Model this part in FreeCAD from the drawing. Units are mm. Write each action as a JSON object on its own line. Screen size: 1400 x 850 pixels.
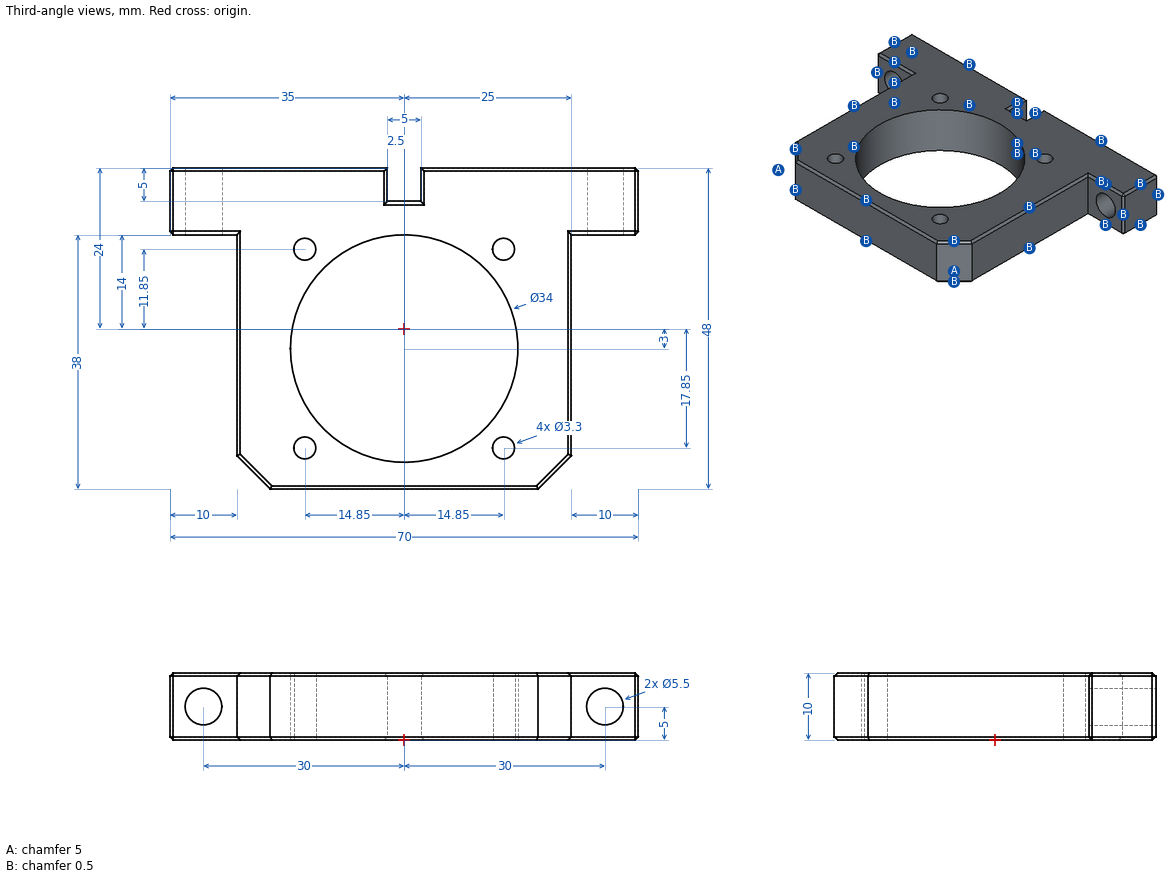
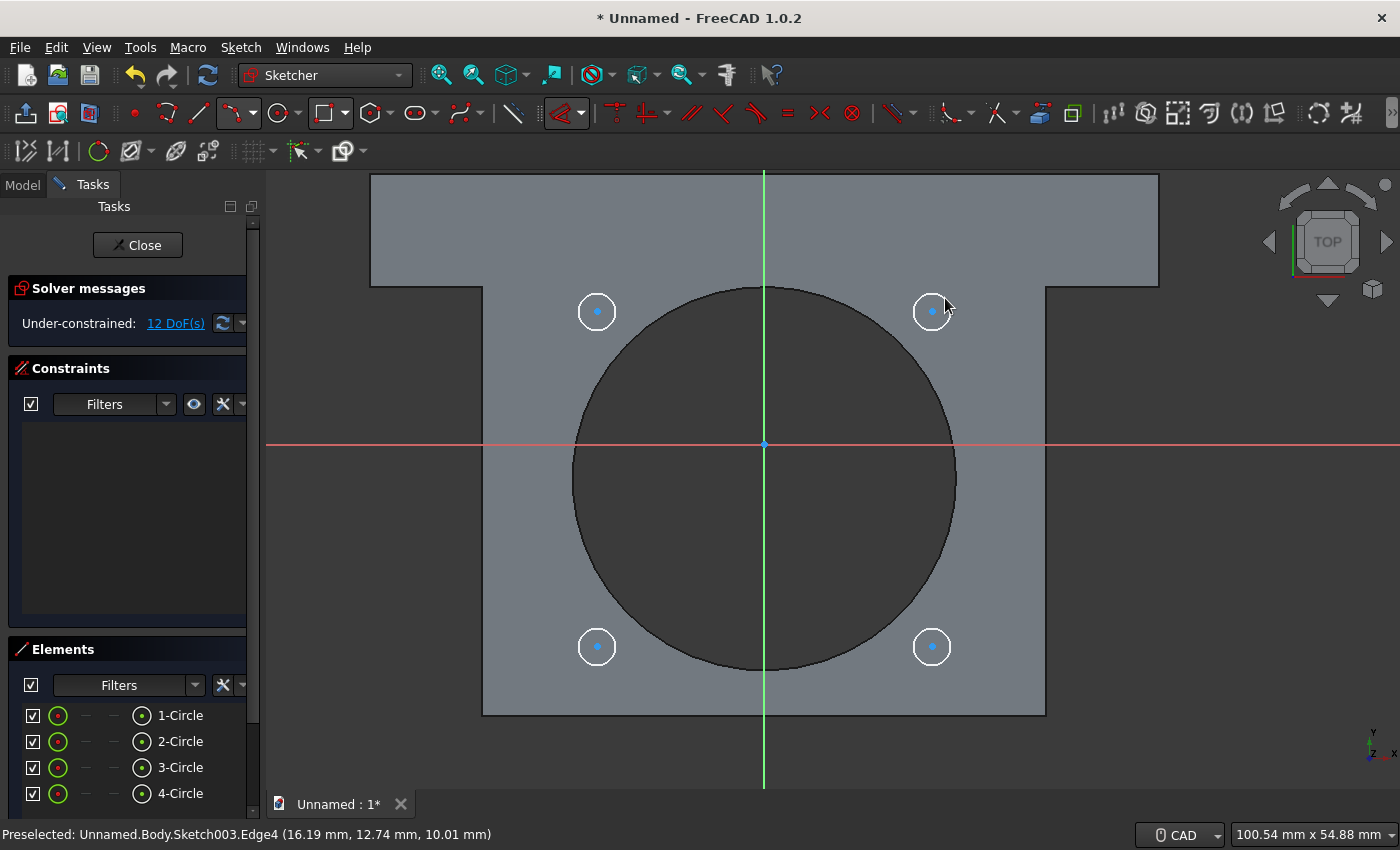
{"action": "left_click", "coordinate": [945, 634]}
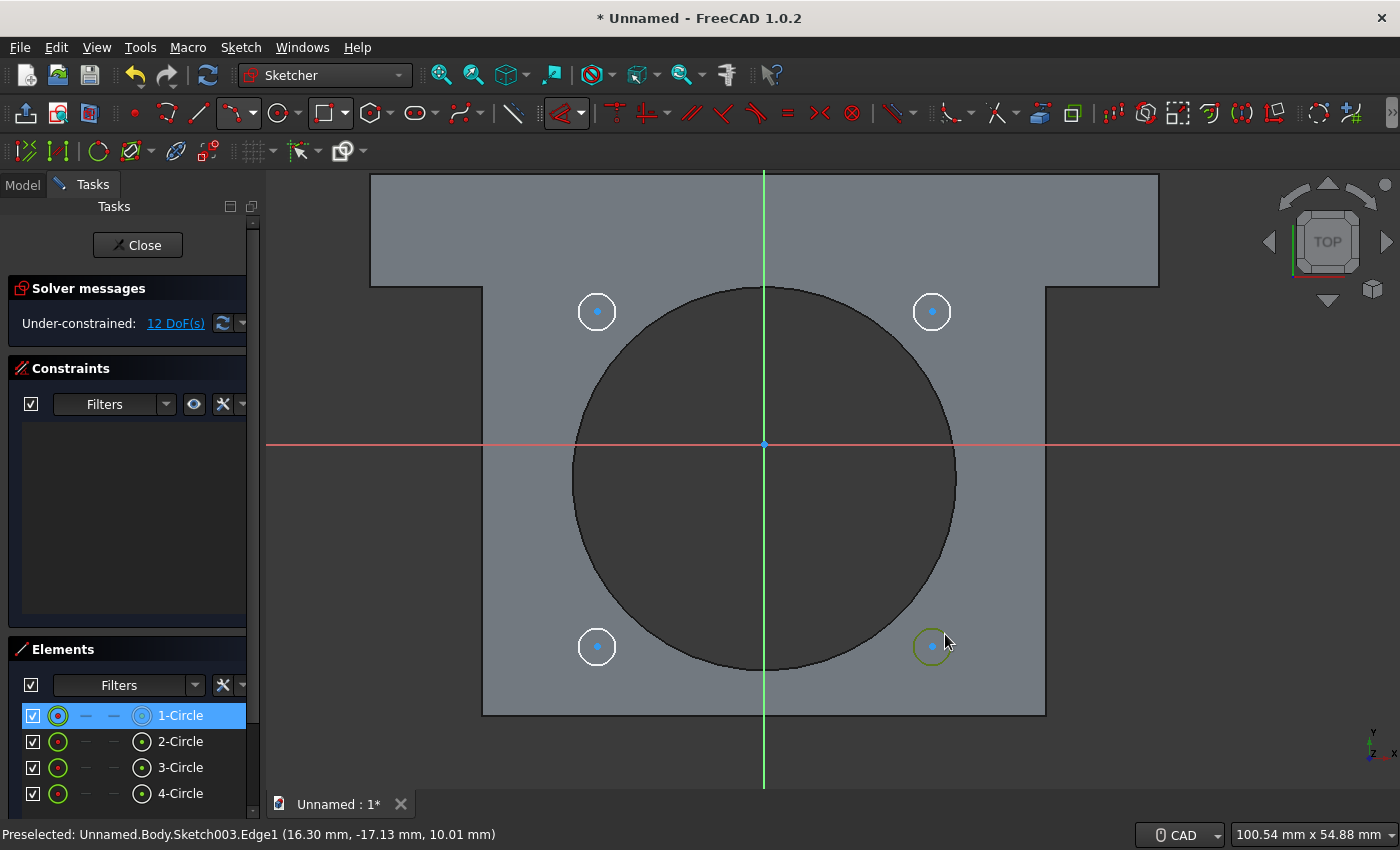
{"action": "left_click", "coordinate": [610, 634]}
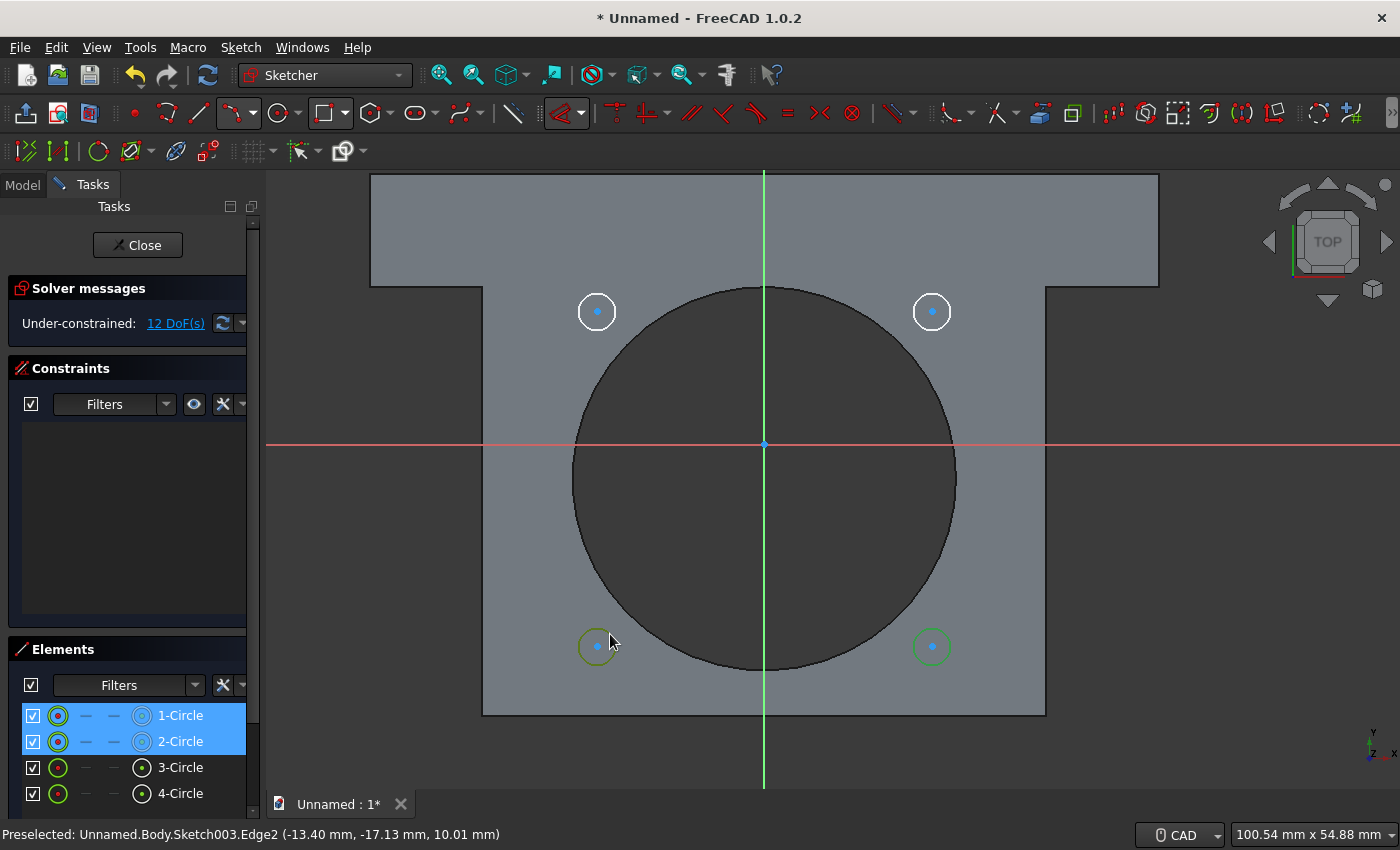
{"action": "left_click", "coordinate": [610, 299]}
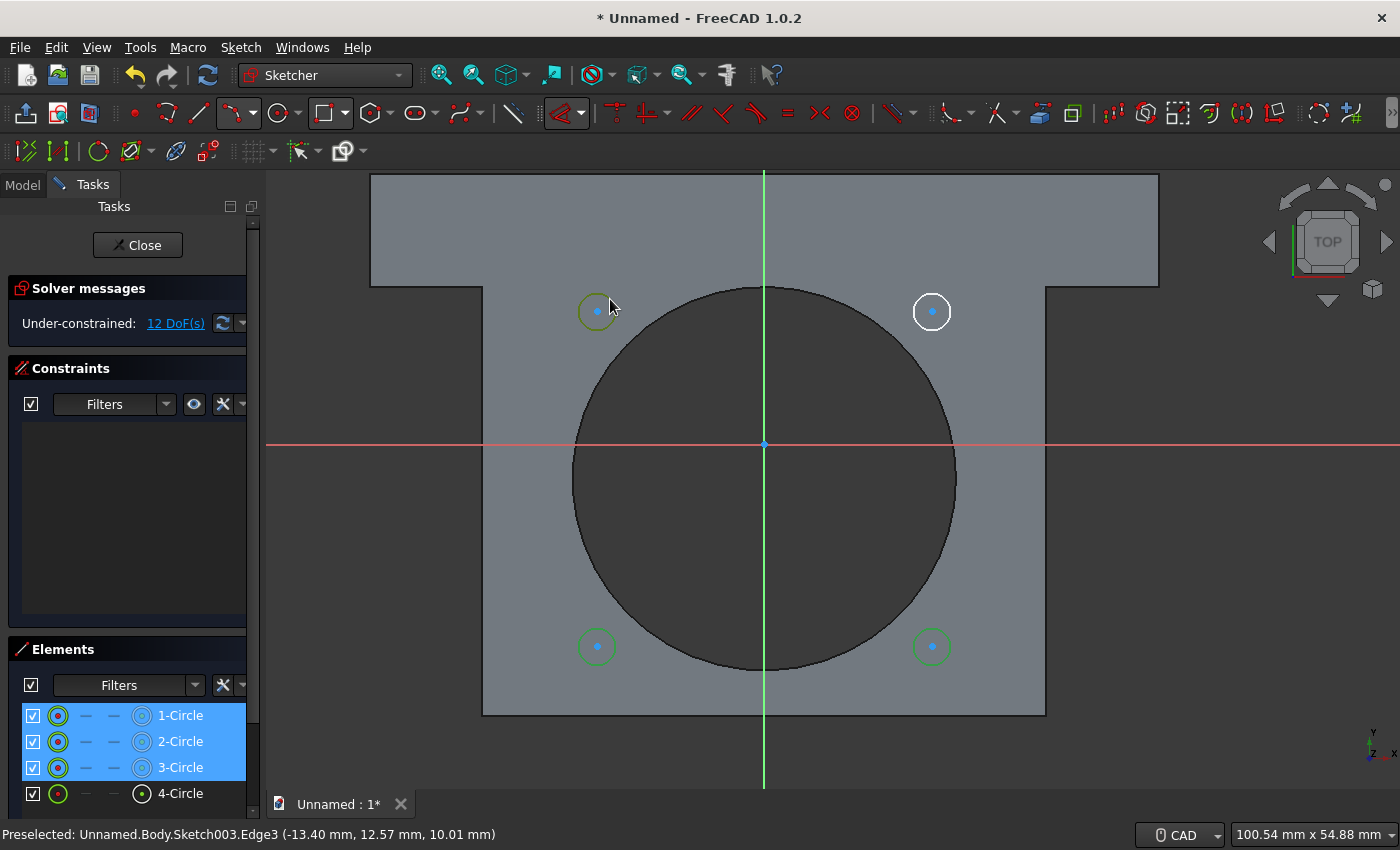
{"action": "left_click", "coordinate": [945, 299]}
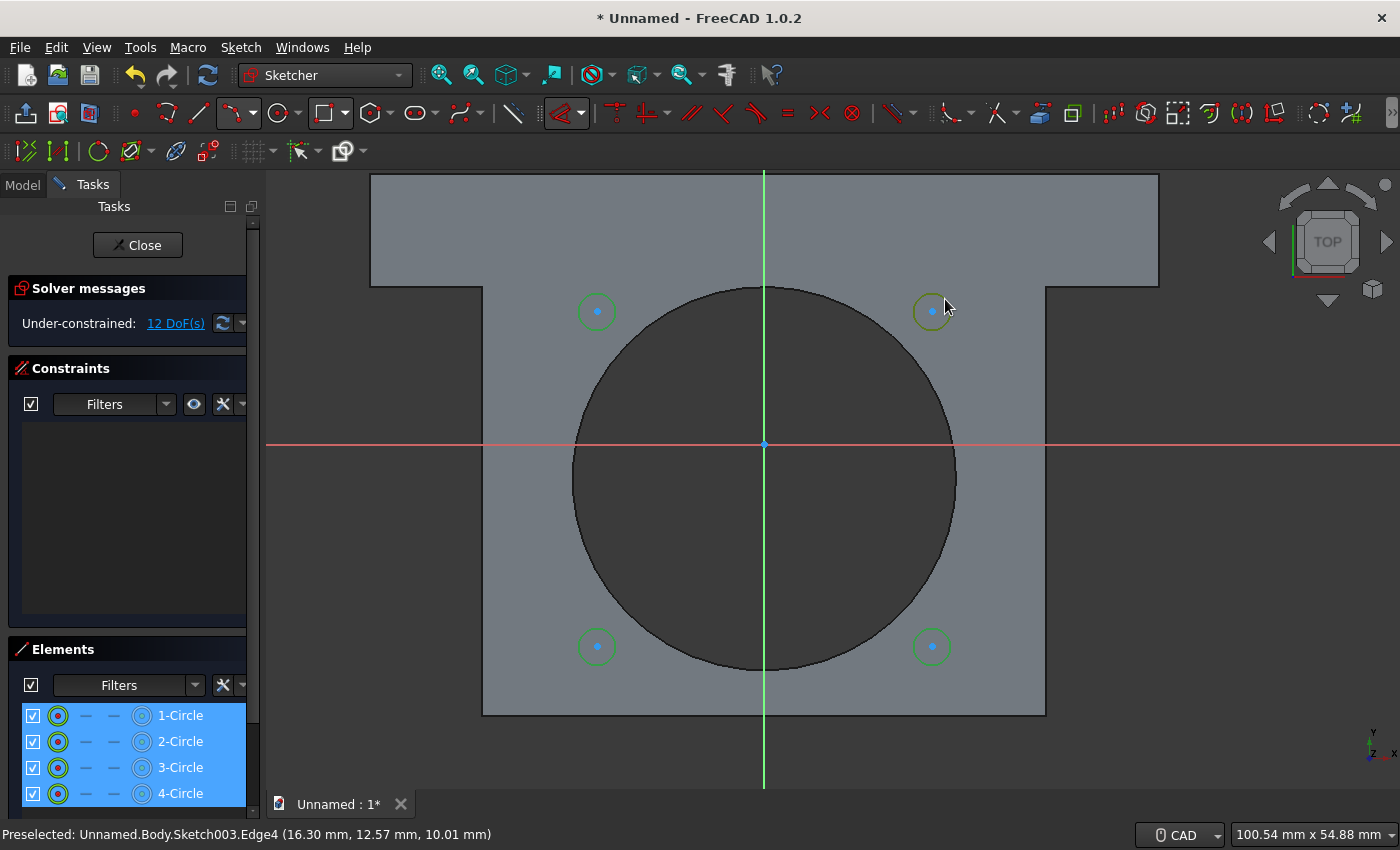
{"action": "left_click", "coordinate": [788, 114]}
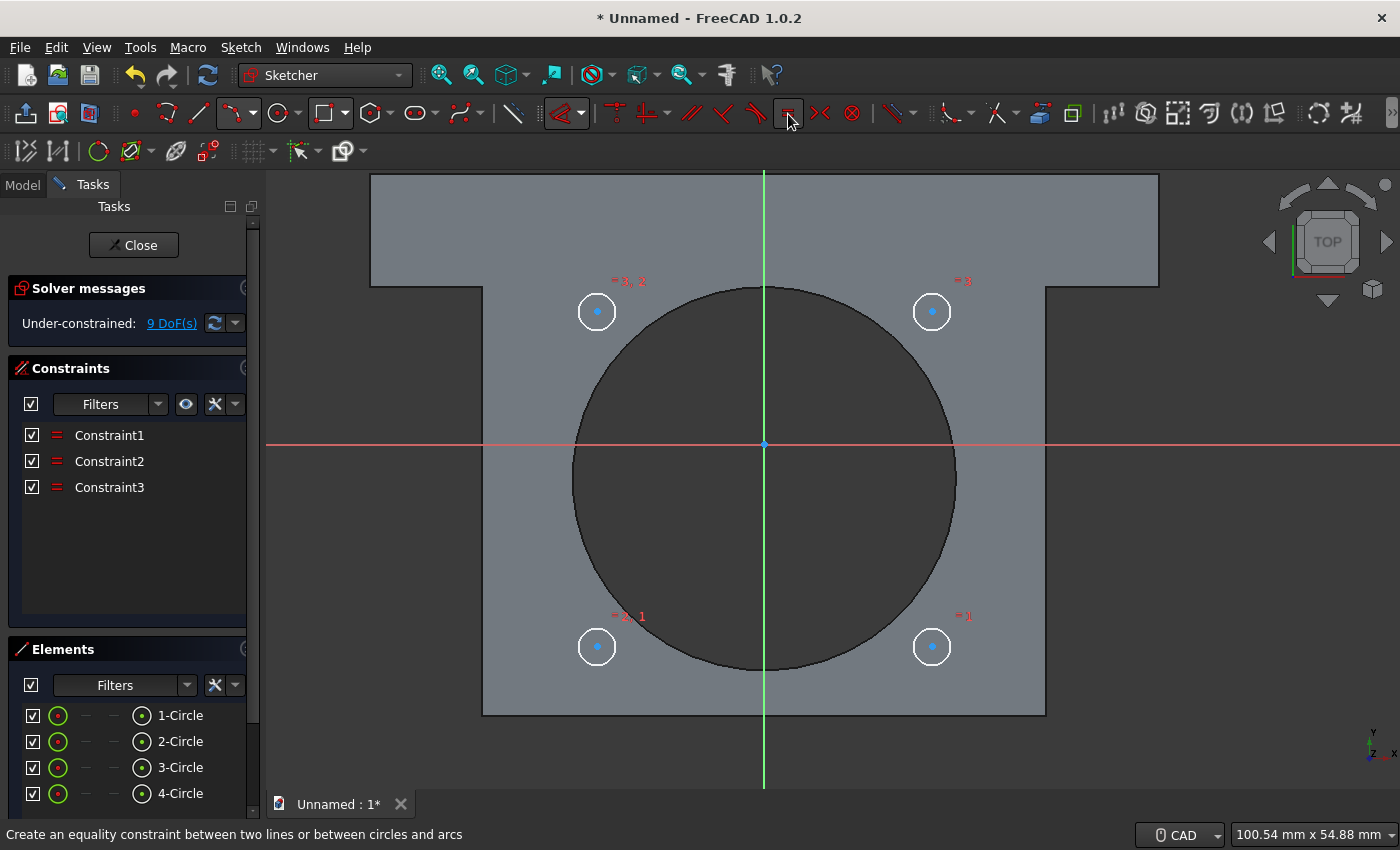
{"action": "left_click", "coordinate": [932, 647]}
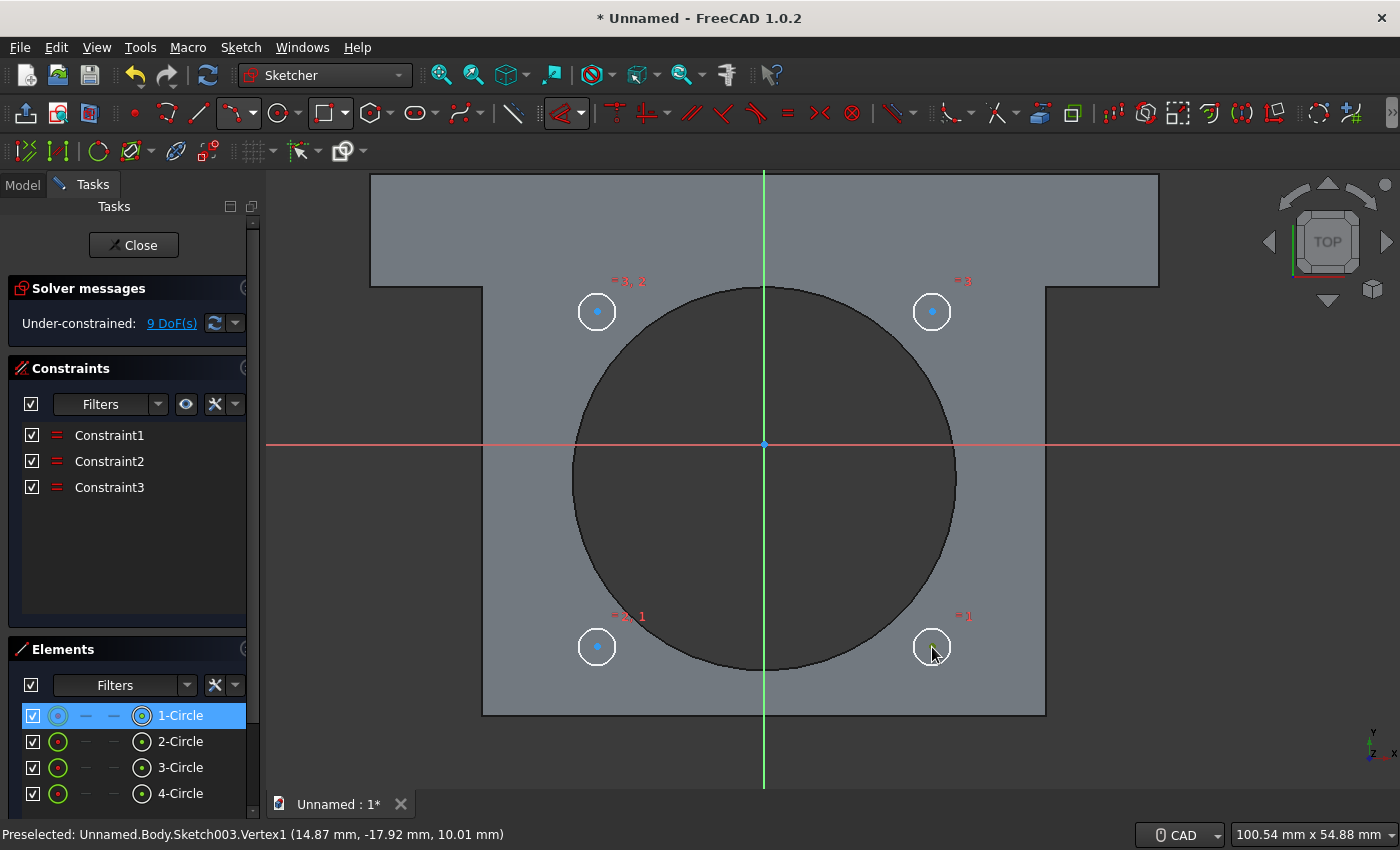
{"action": "left_click", "coordinate": [597, 647]}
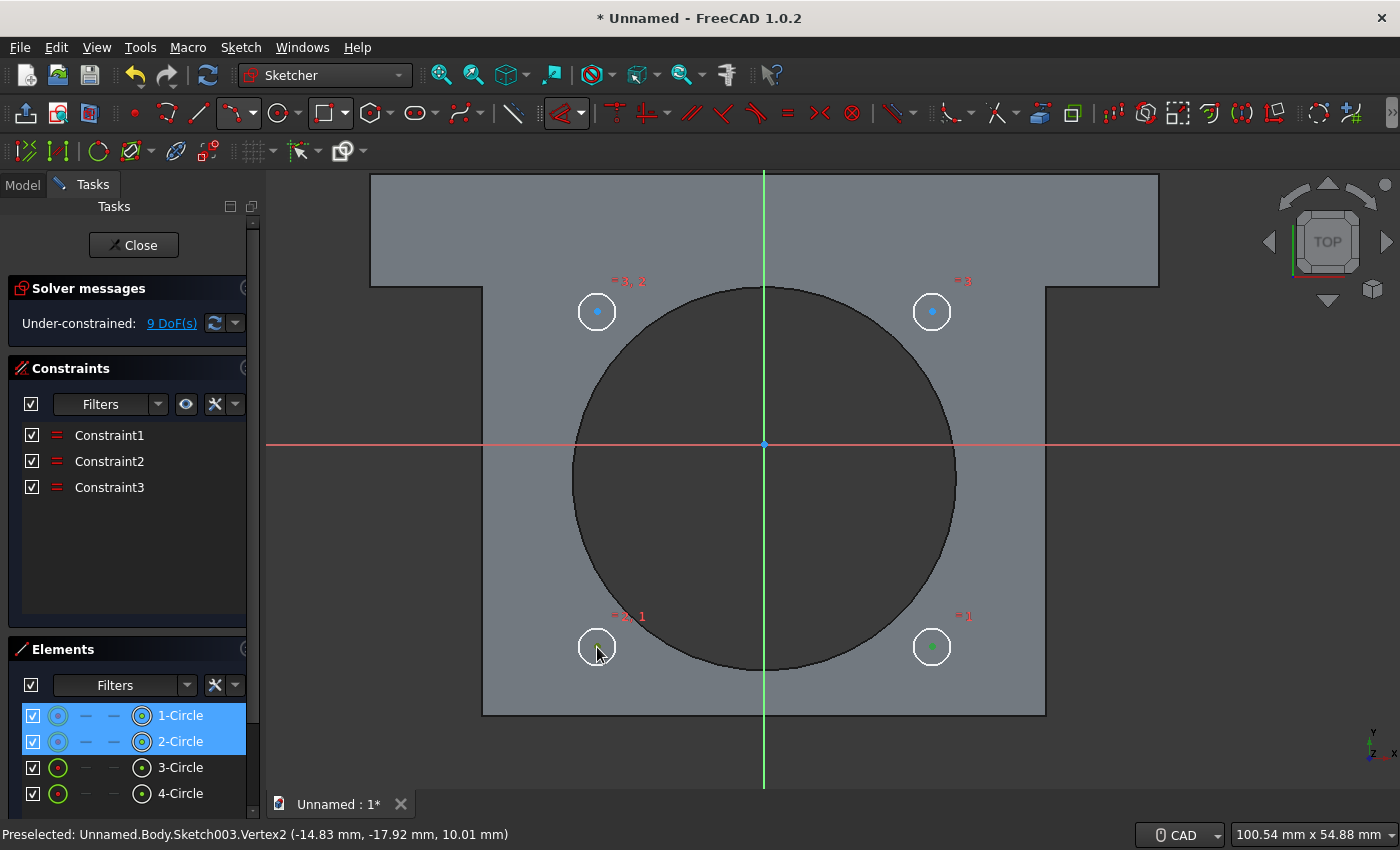
{"action": "left_click", "coordinate": [670, 114]}